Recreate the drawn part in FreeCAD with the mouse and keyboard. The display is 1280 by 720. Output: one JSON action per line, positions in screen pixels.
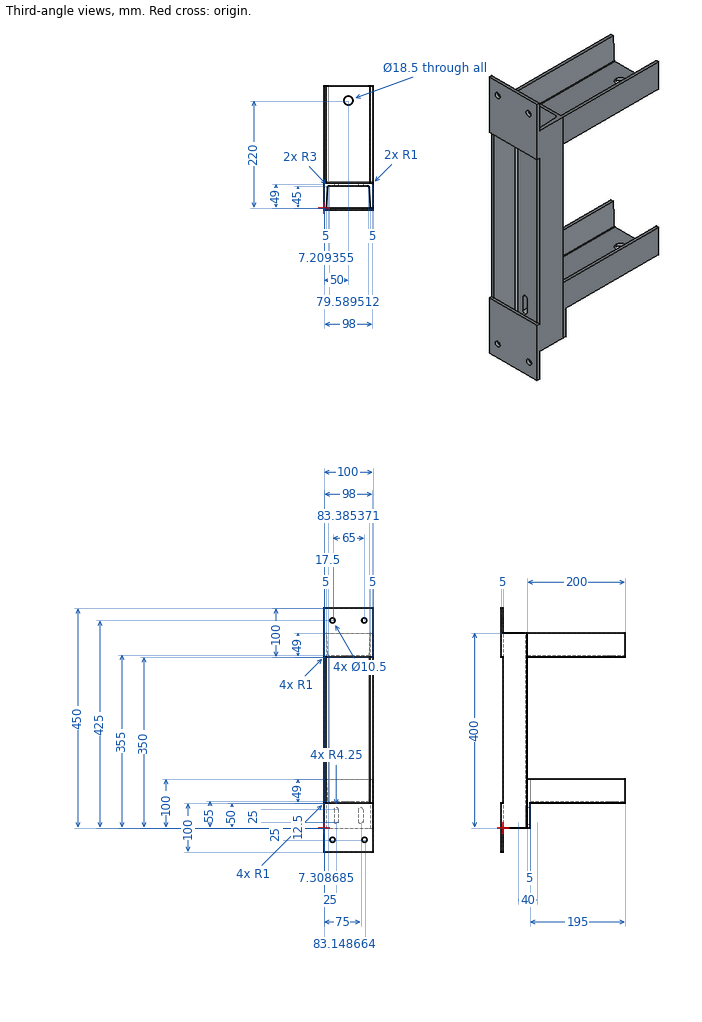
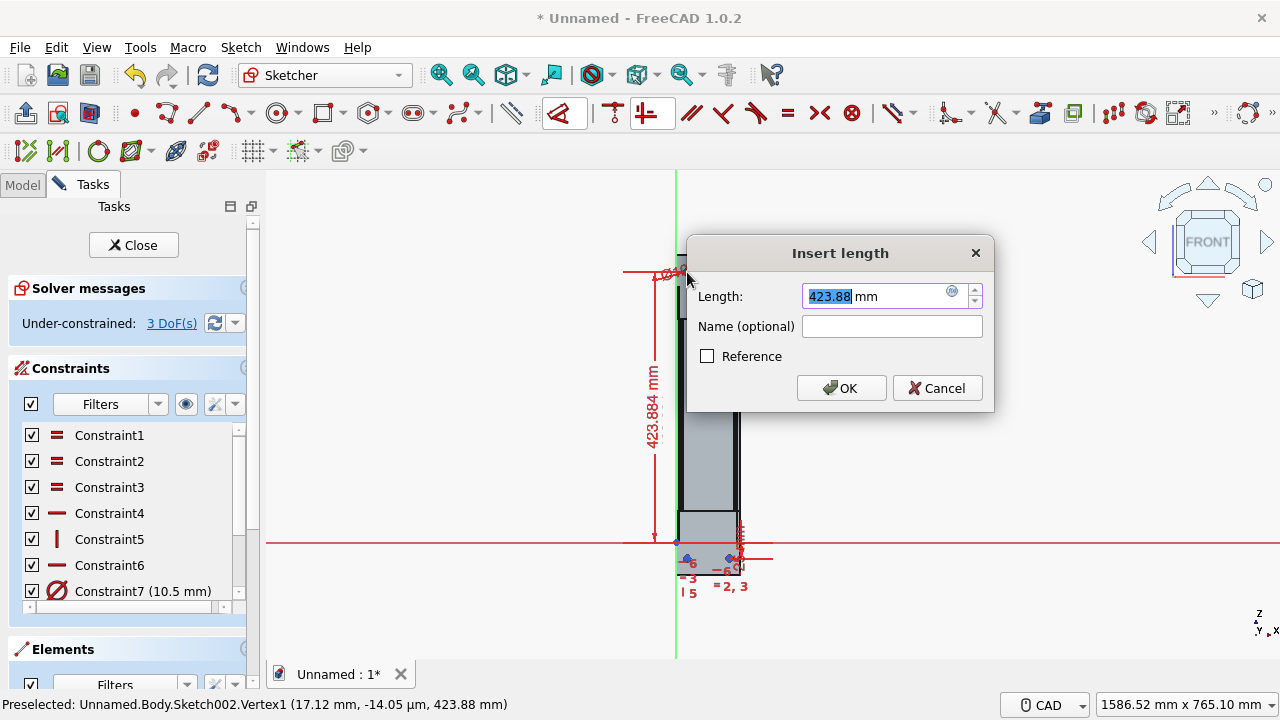
{"action": "type", "text": "425"}
{"action": "key", "text": "Return"}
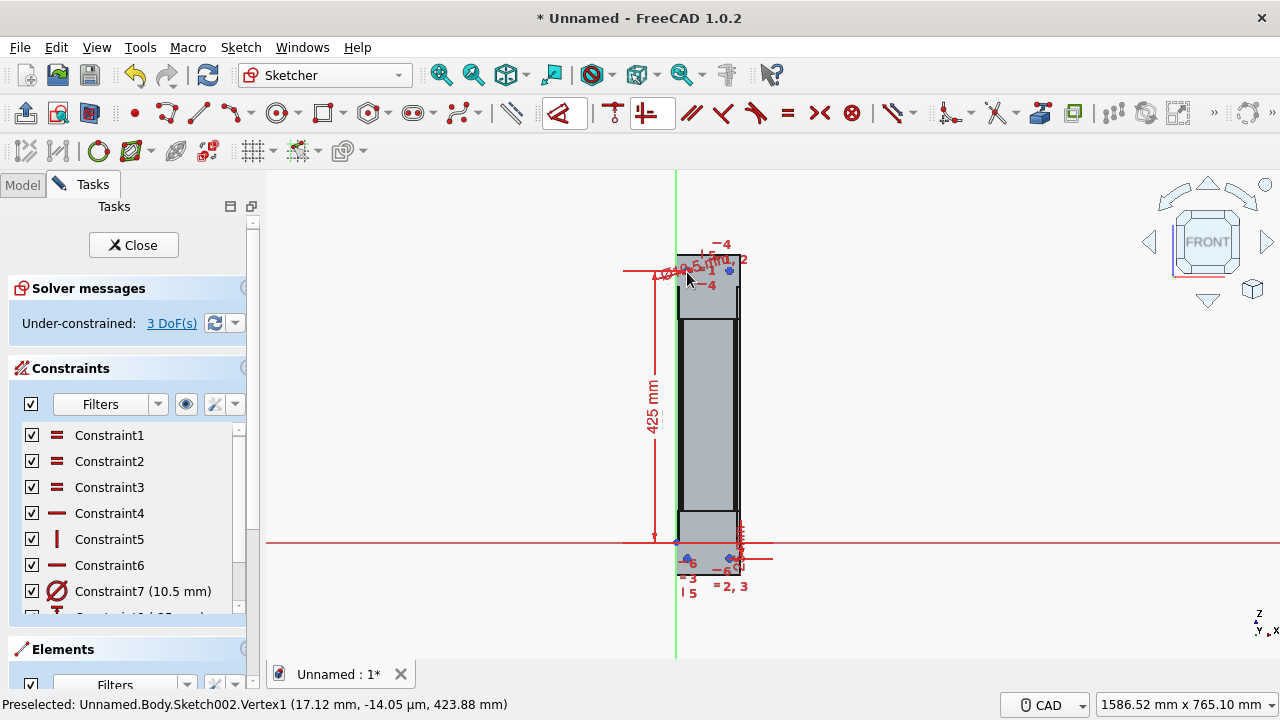
{"action": "left_click", "coordinate": [687, 271]}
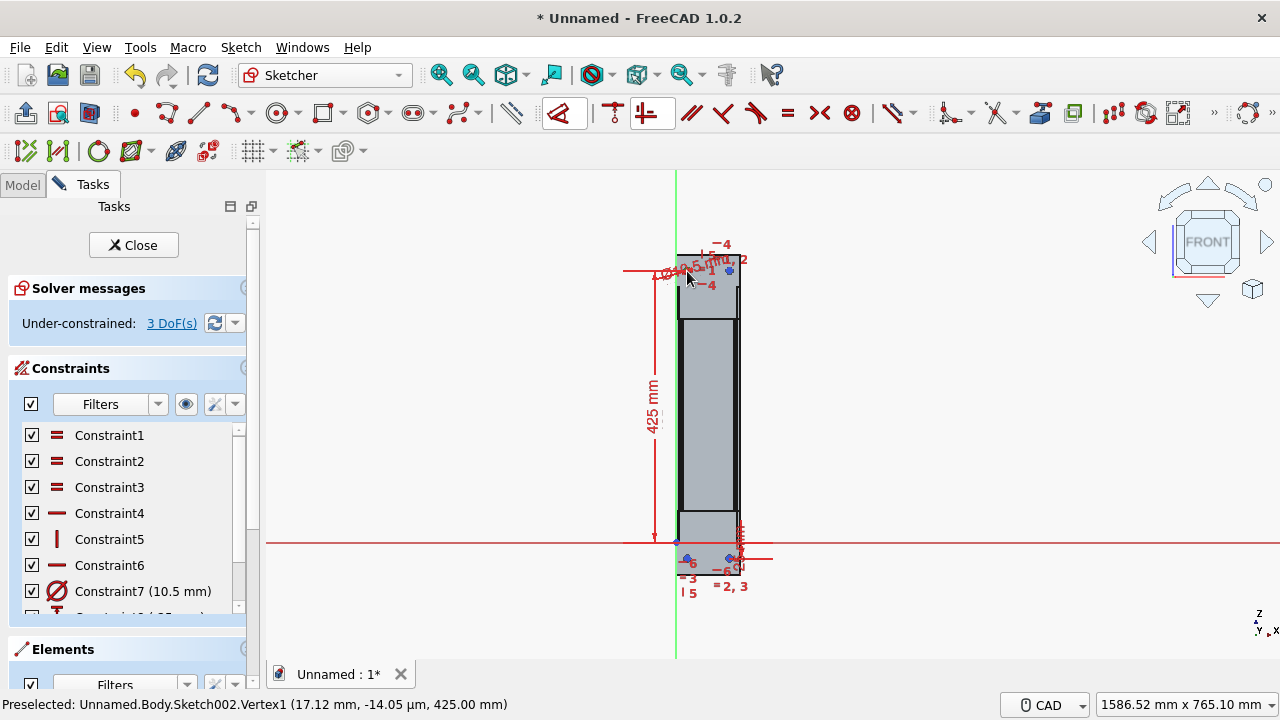
{"action": "left_click", "coordinate": [730, 271]}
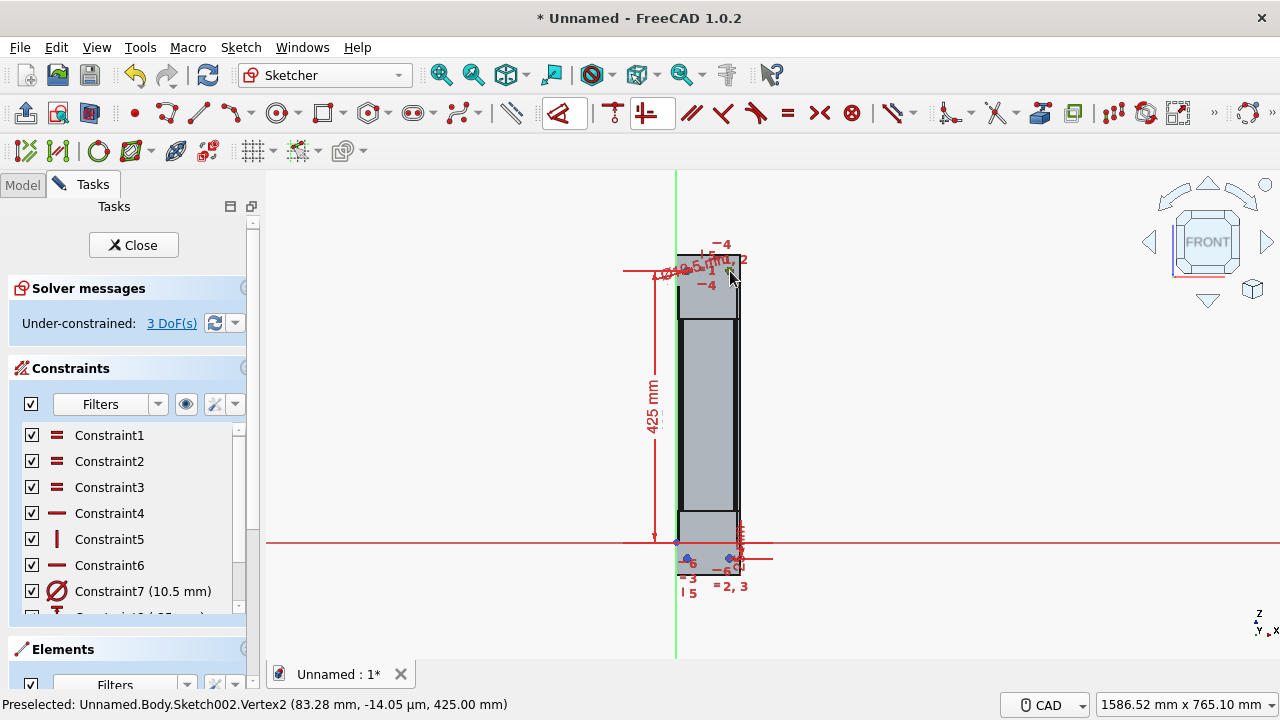
{"action": "key", "text": "l"}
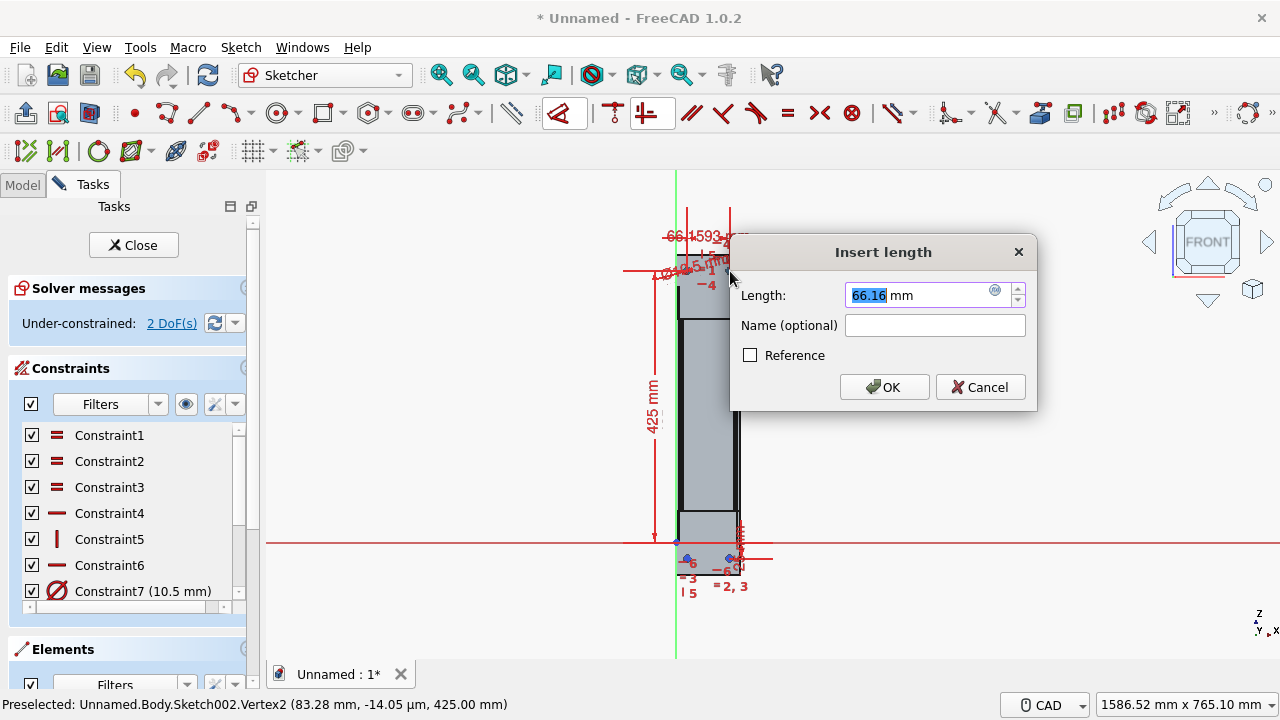
{"action": "type", "text": "65"}
{"action": "key", "text": "Return"}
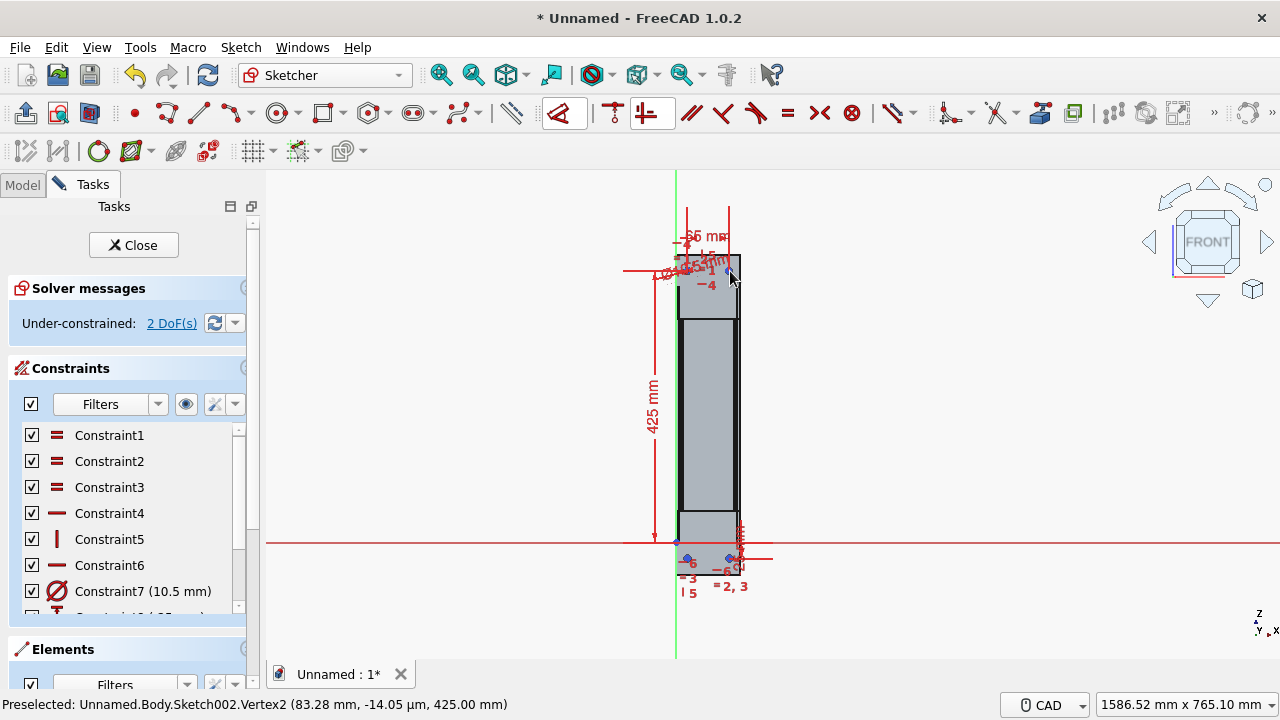
{"action": "scroll", "coordinate": [687, 271], "scroll_direction": "up", "scroll_amount": 7}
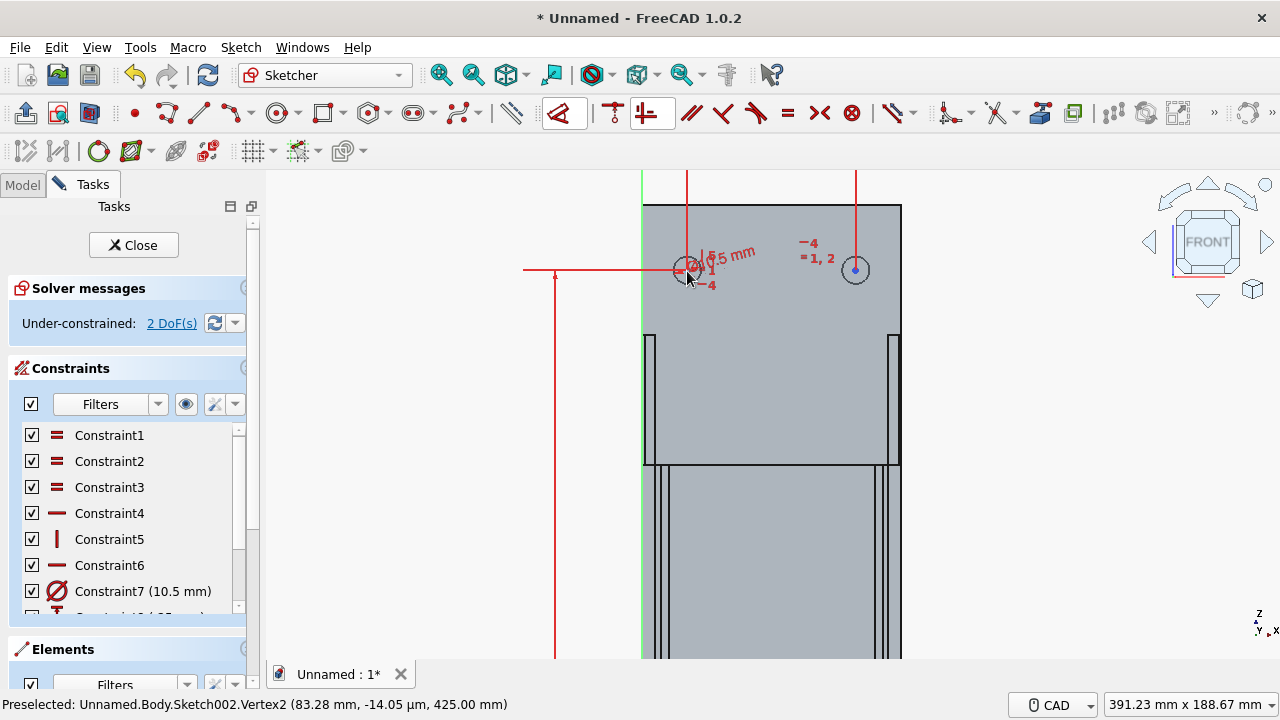
{"action": "left_click", "coordinate": [687, 270]}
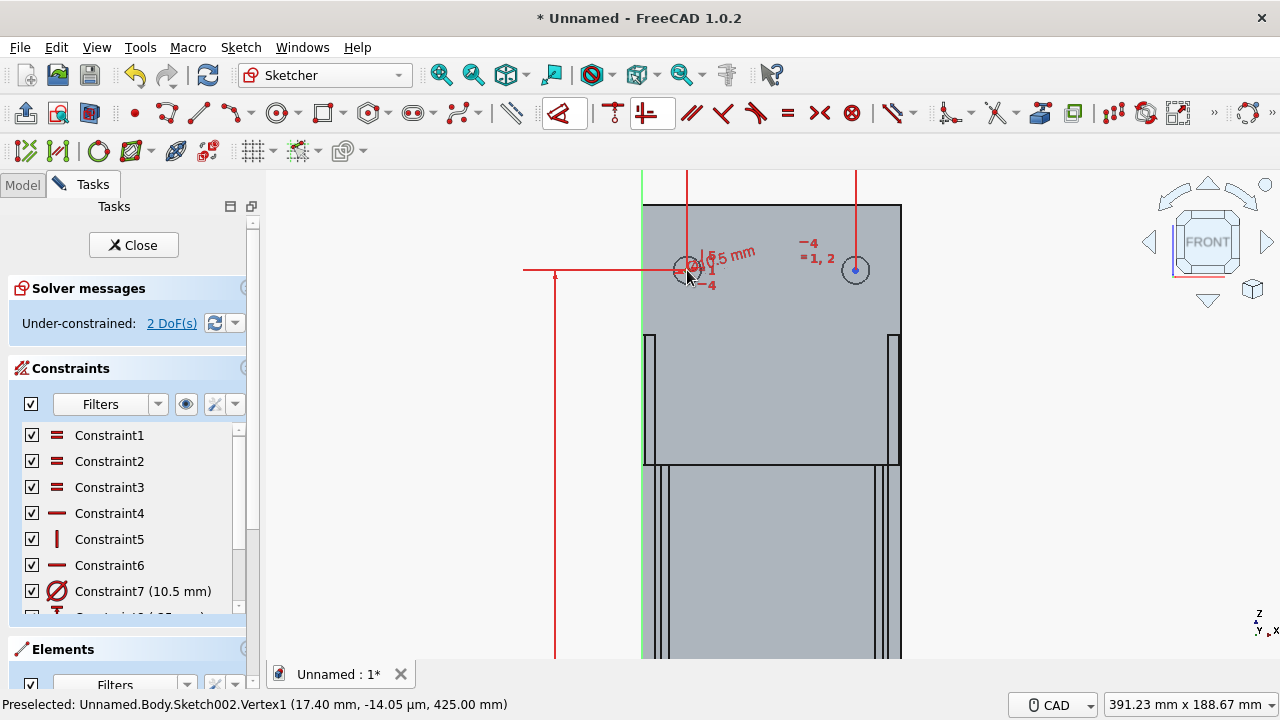
{"action": "key", "text": "l"}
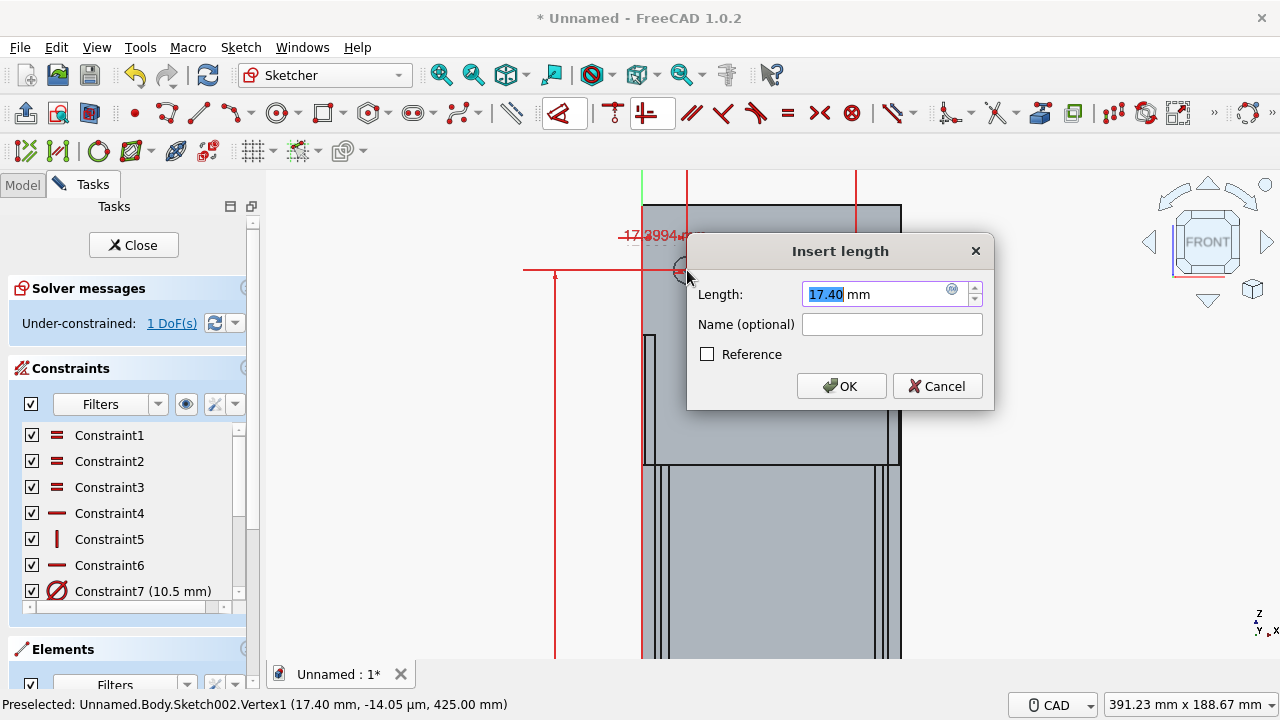
{"action": "type", "text": "17.5"}
{"action": "key", "text": "Return"}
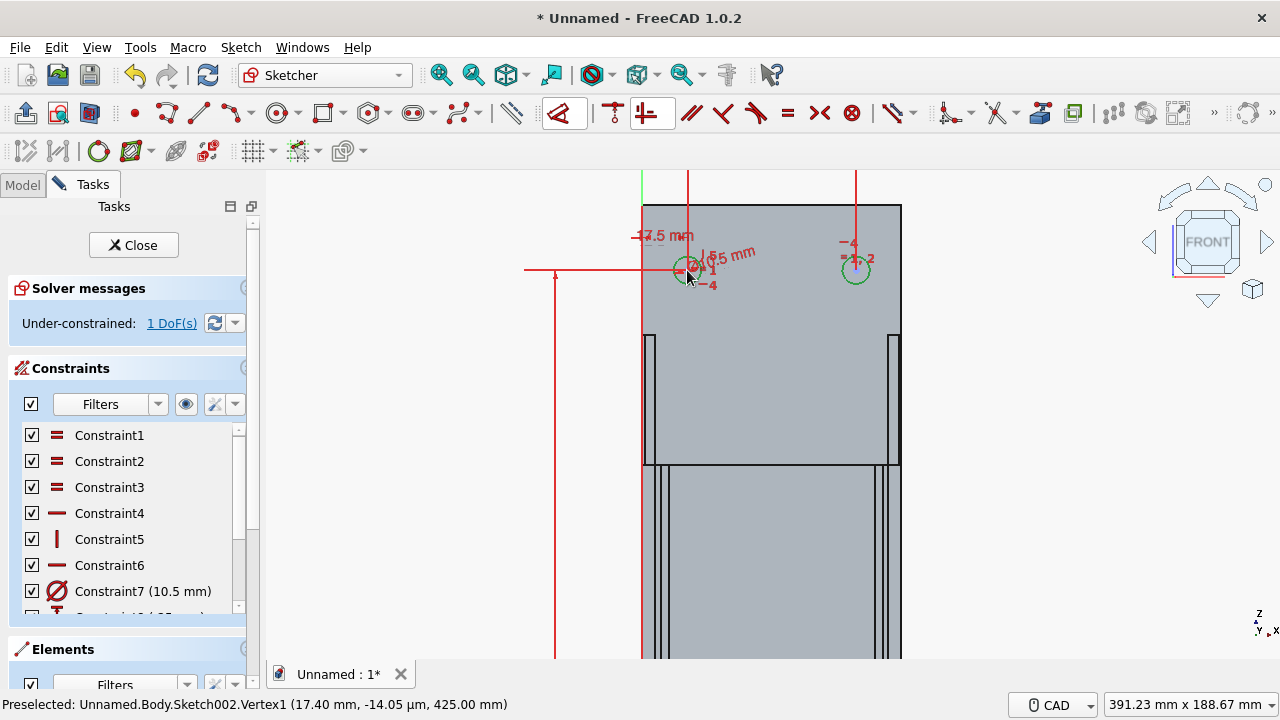
{"action": "scroll", "coordinate": [687, 271], "scroll_direction": "down", "scroll_amount": 7}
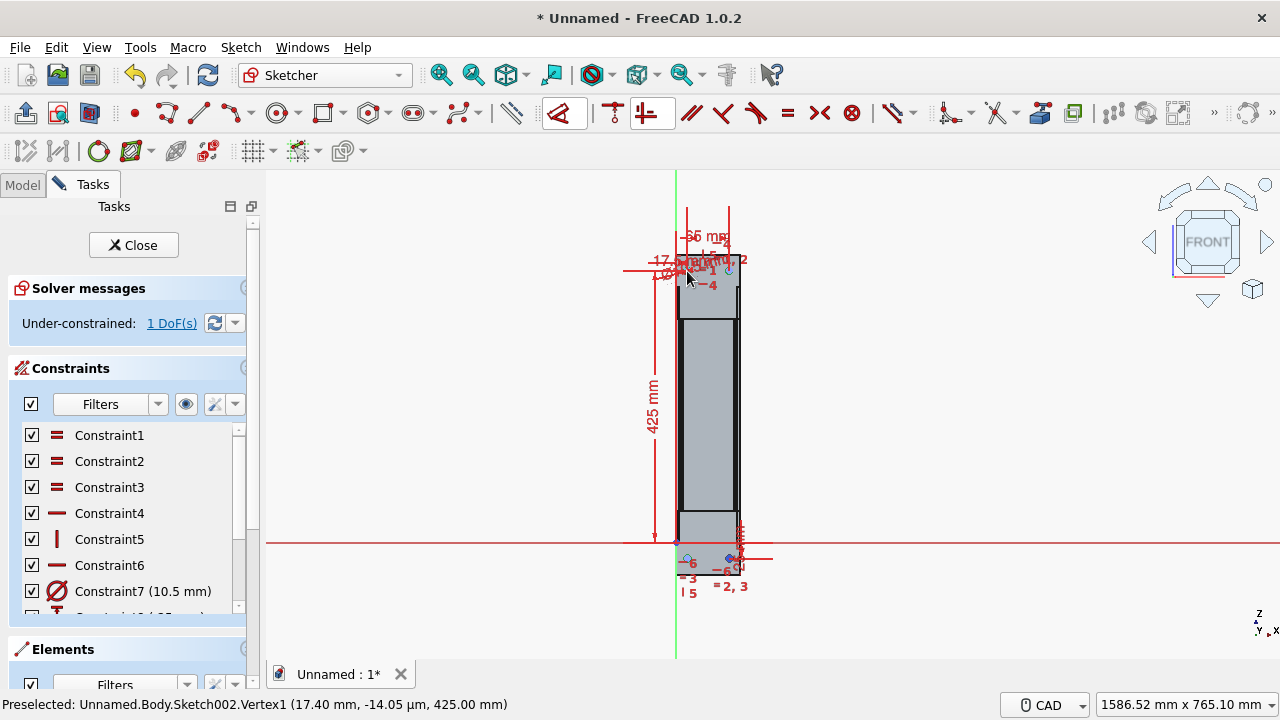
{"action": "left_click", "coordinate": [730, 559]}